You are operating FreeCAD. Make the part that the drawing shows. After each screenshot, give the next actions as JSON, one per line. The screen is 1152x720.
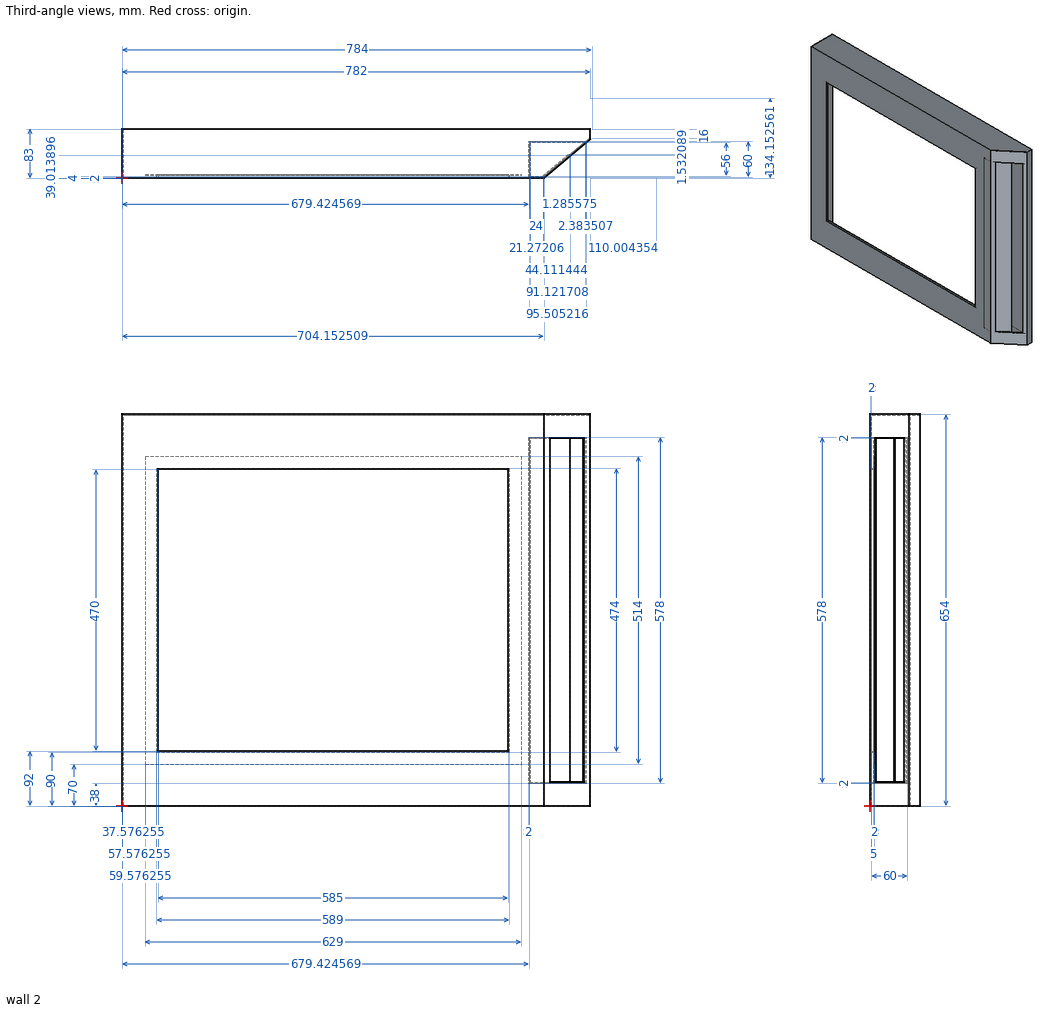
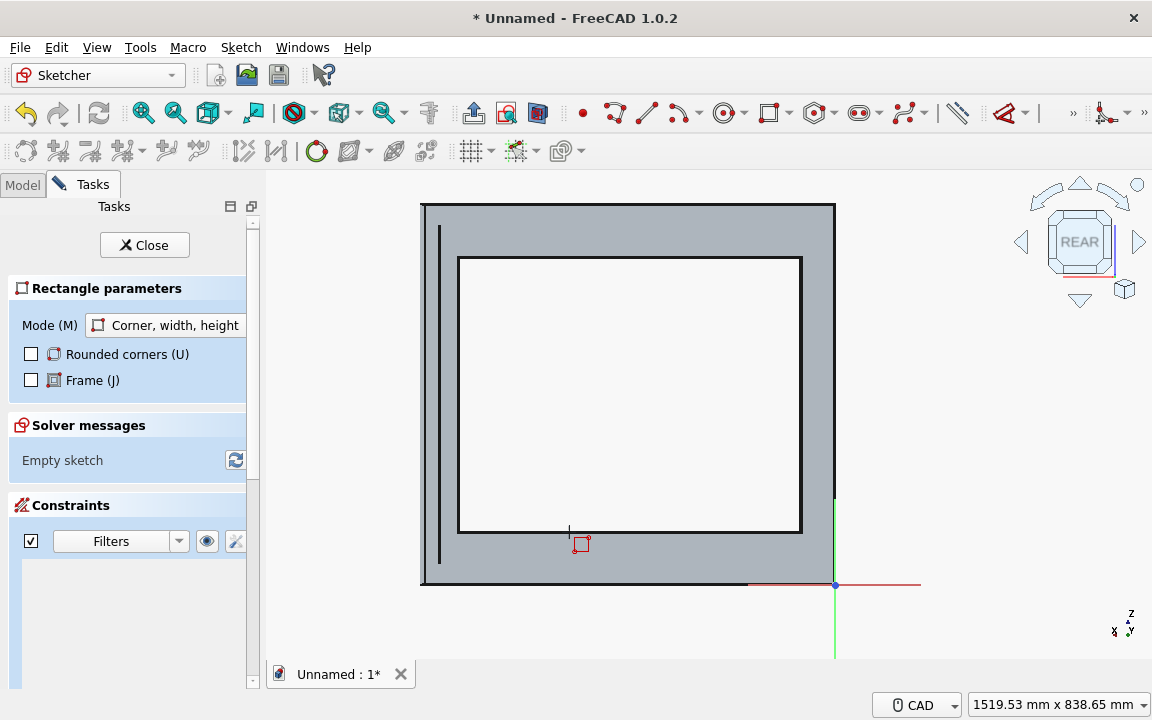
{"action": "left_click", "coordinate": [446, 245]}
{"action": "left_click", "coordinate": [813, 545]}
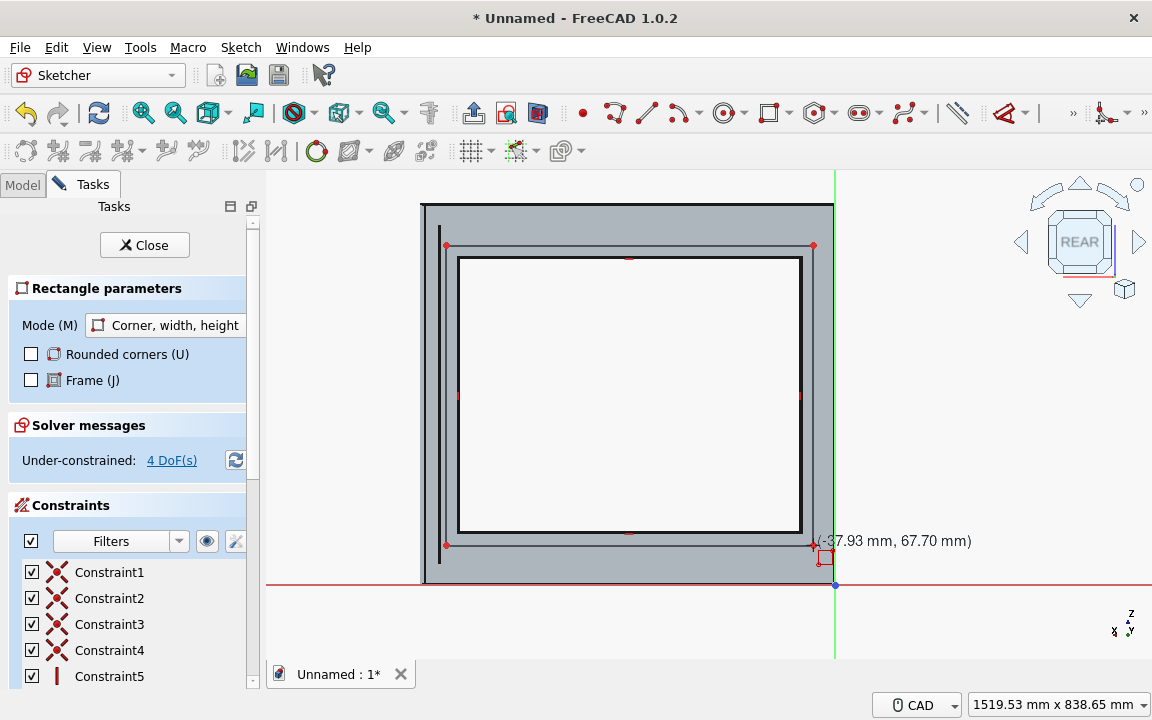
{"action": "scroll", "coordinate": [459, 258], "scroll_direction": "up", "scroll_amount": 2}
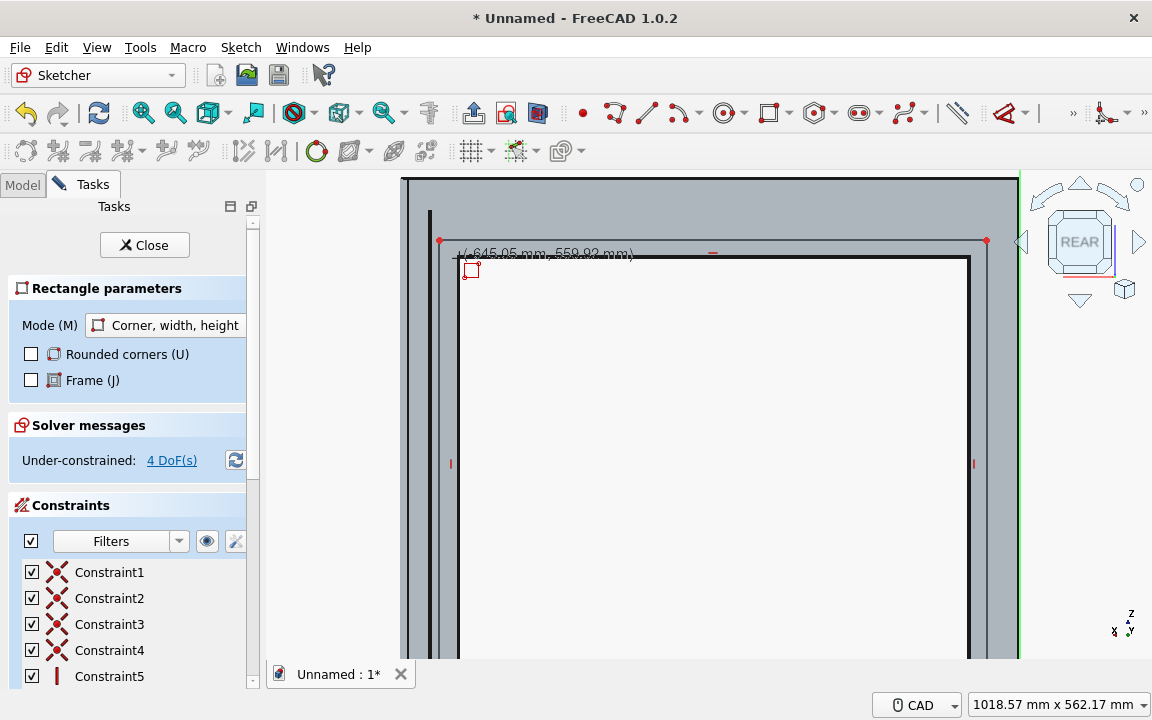
{"action": "left_click", "coordinate": [459, 258]}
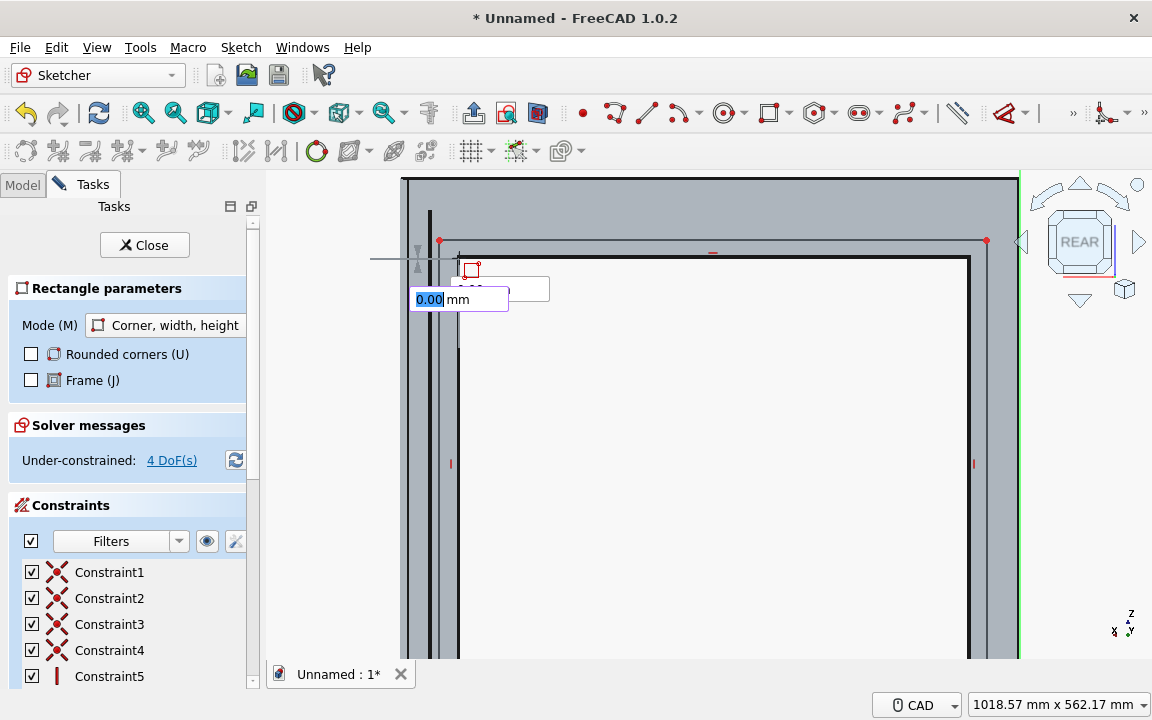
{"action": "scroll", "coordinate": [532, 320], "scroll_direction": "down", "scroll_amount": 3}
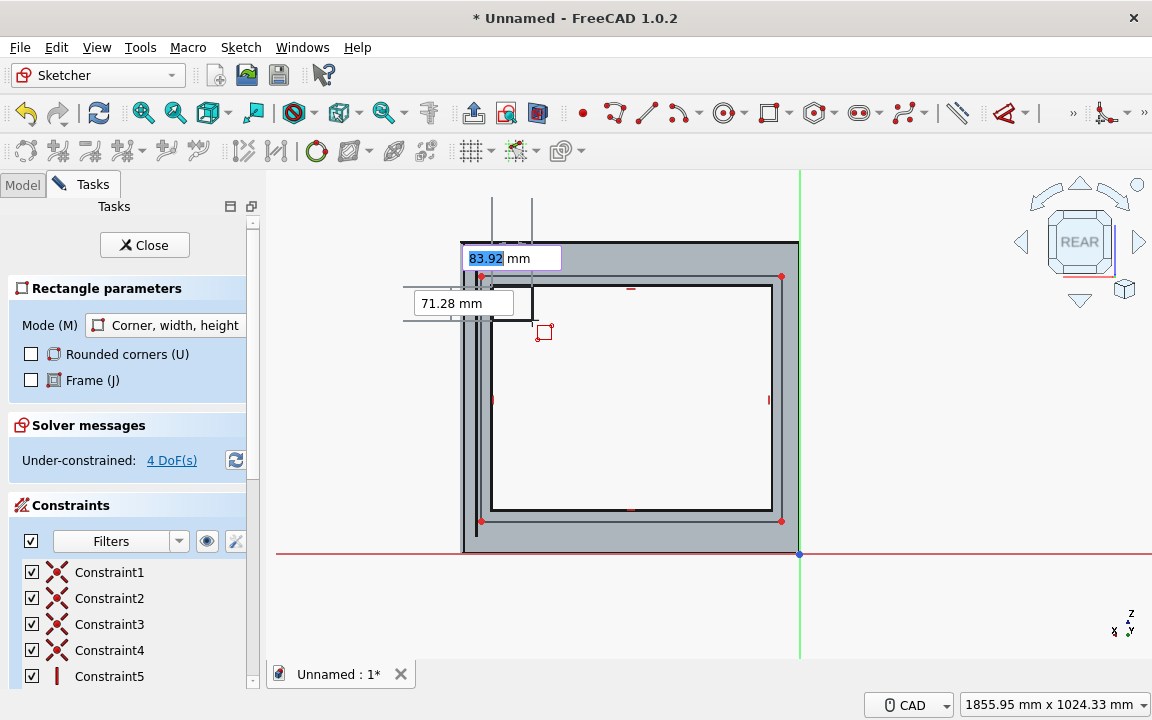
{"action": "scroll", "coordinate": [772, 510], "scroll_direction": "up", "scroll_amount": 3}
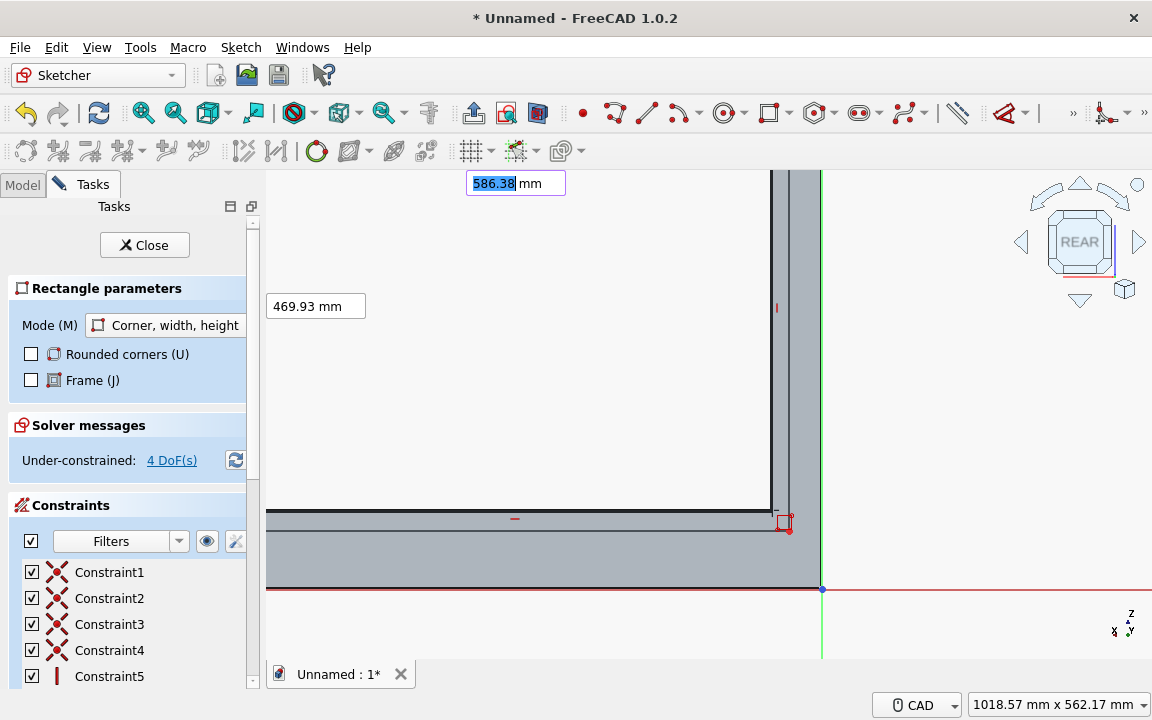
{"action": "left_click", "coordinate": [771, 510]}
{"action": "key", "text": "Escape"}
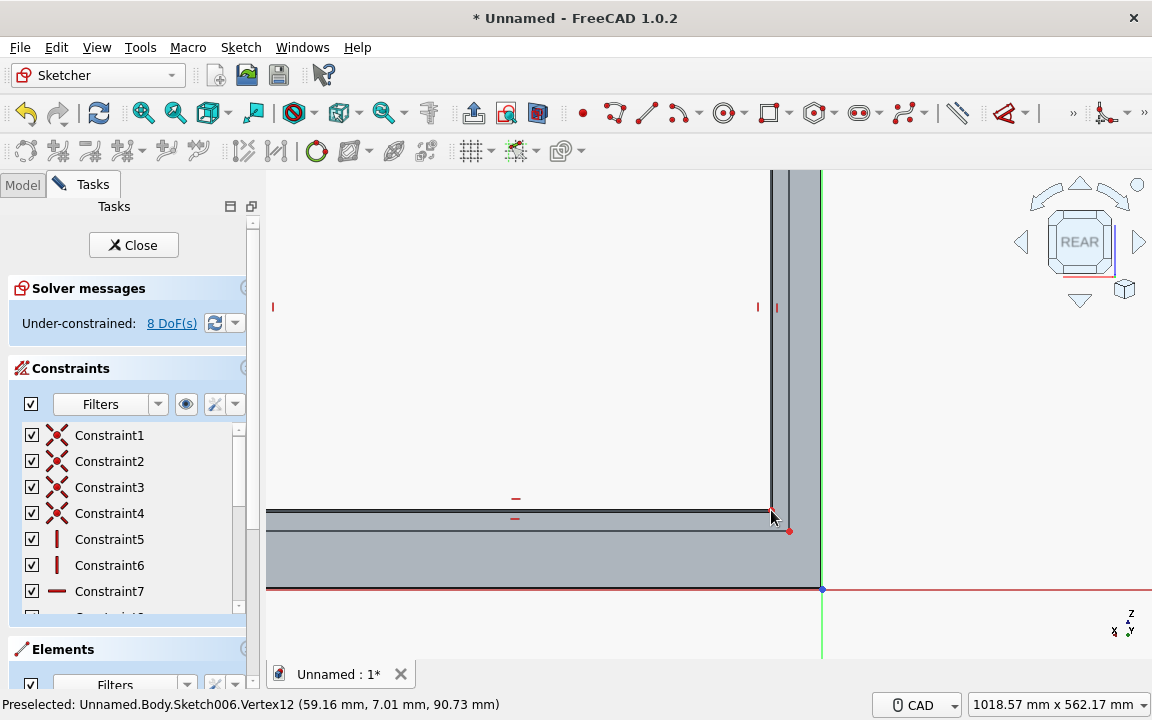
{"action": "left_click", "coordinate": [1004, 114]}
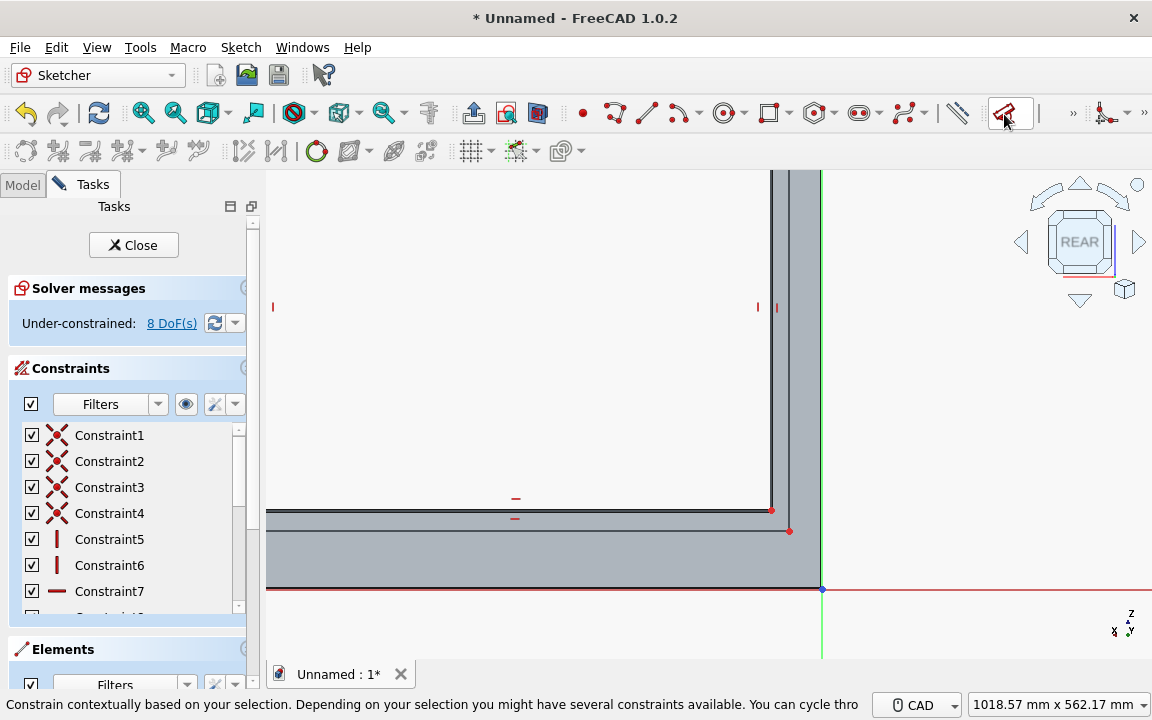
{"action": "scroll", "coordinate": [772, 510], "scroll_direction": "down", "scroll_amount": 3}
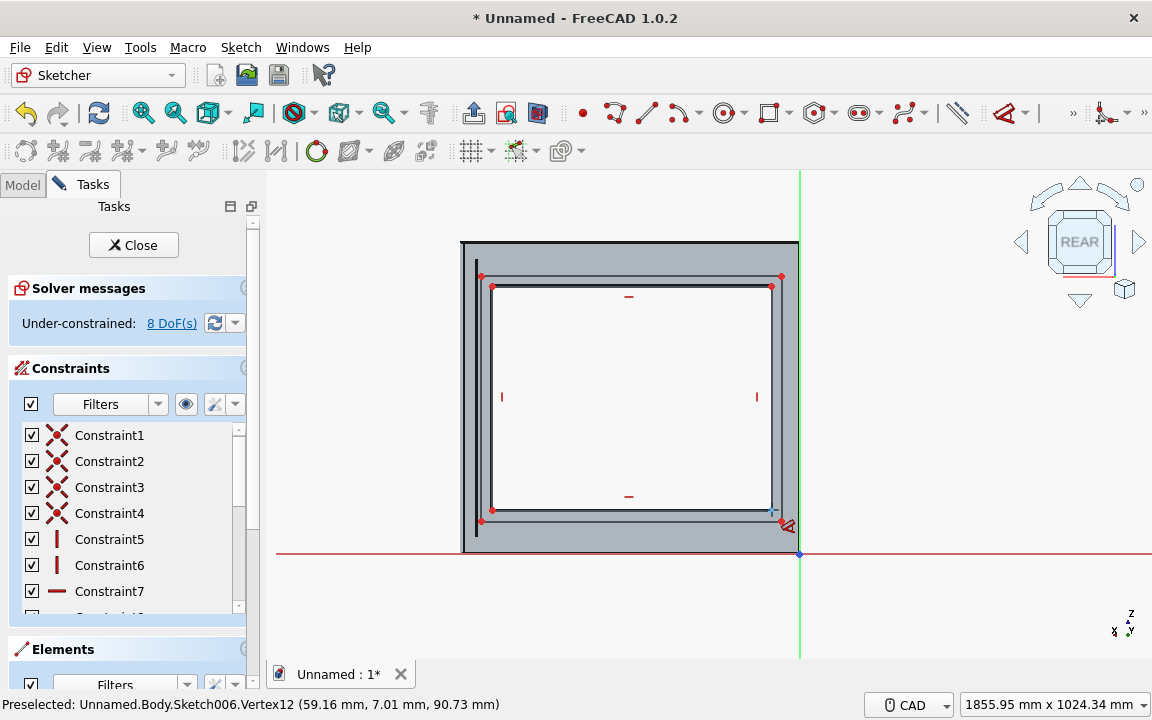
{"action": "scroll", "coordinate": [481, 350], "scroll_direction": "up", "scroll_amount": 2}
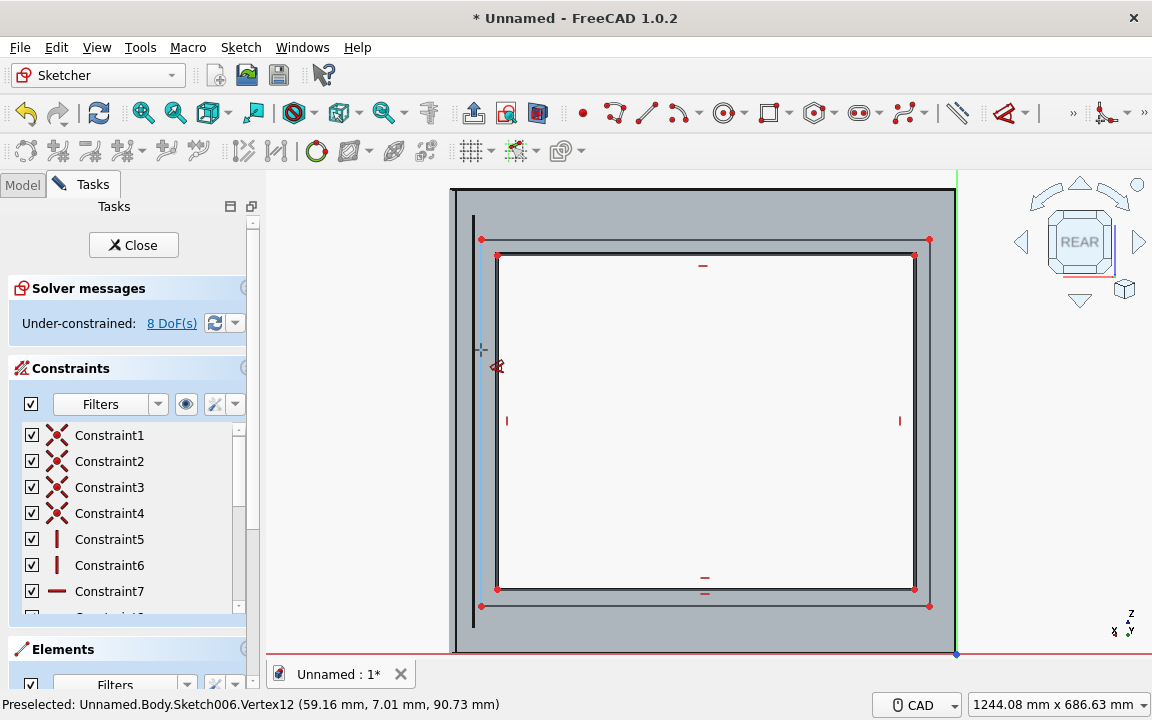
{"action": "left_click", "coordinate": [481, 350]}
{"action": "left_click", "coordinate": [447, 423]}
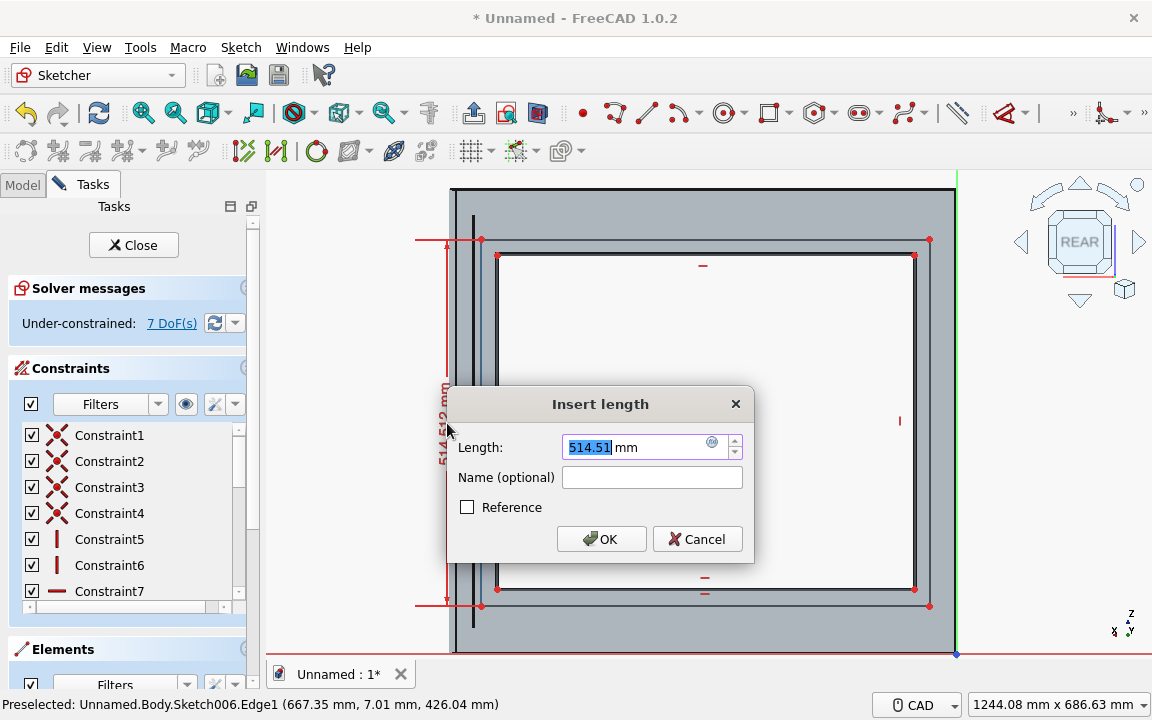
{"action": "type", "text": "514"}
{"action": "key", "text": "Return"}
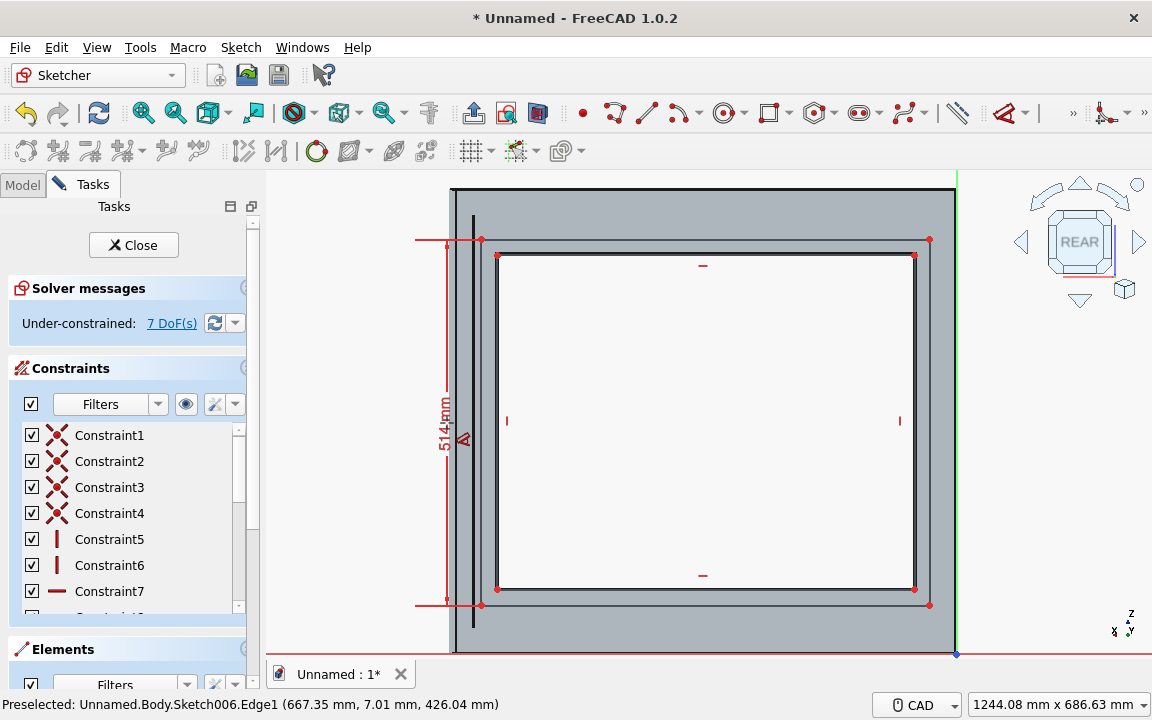
{"action": "left_click", "coordinate": [616, 606]}
{"action": "left_click", "coordinate": [706, 572]}